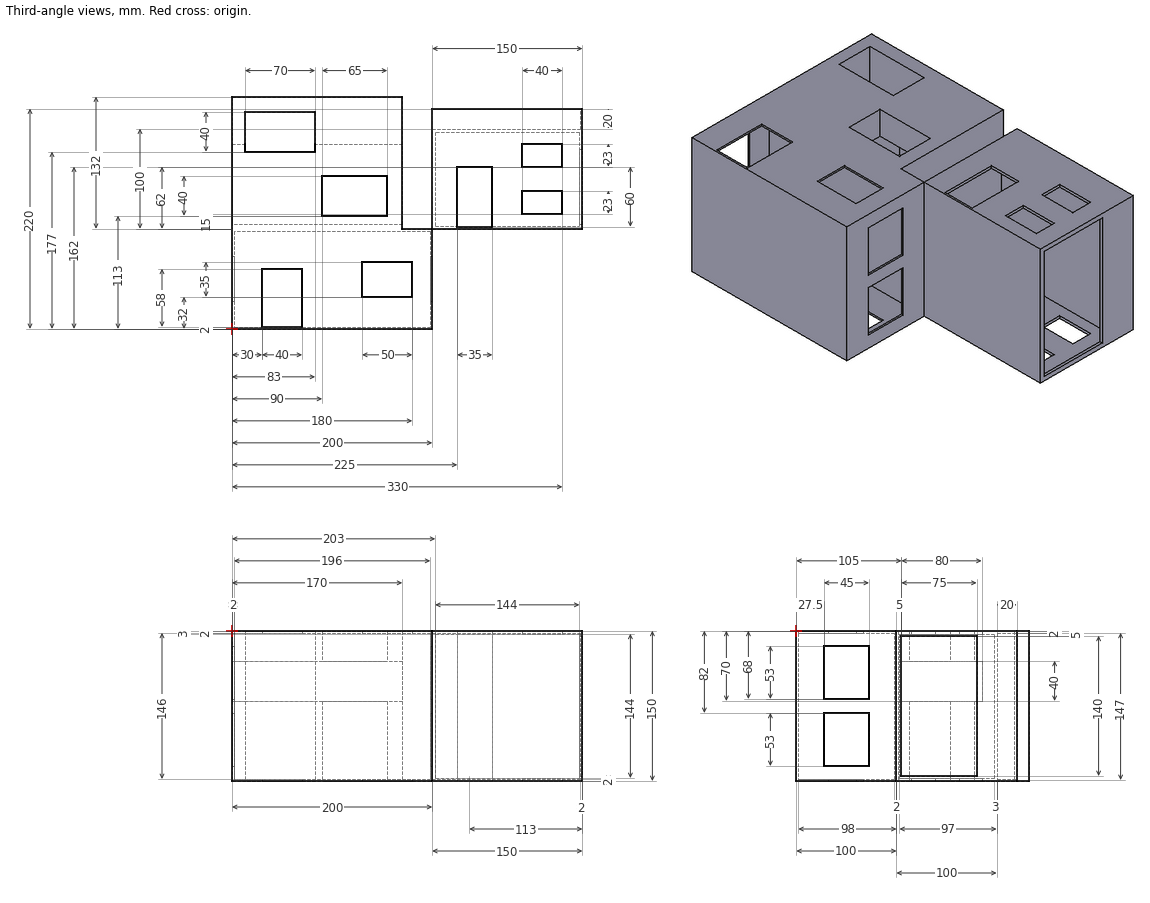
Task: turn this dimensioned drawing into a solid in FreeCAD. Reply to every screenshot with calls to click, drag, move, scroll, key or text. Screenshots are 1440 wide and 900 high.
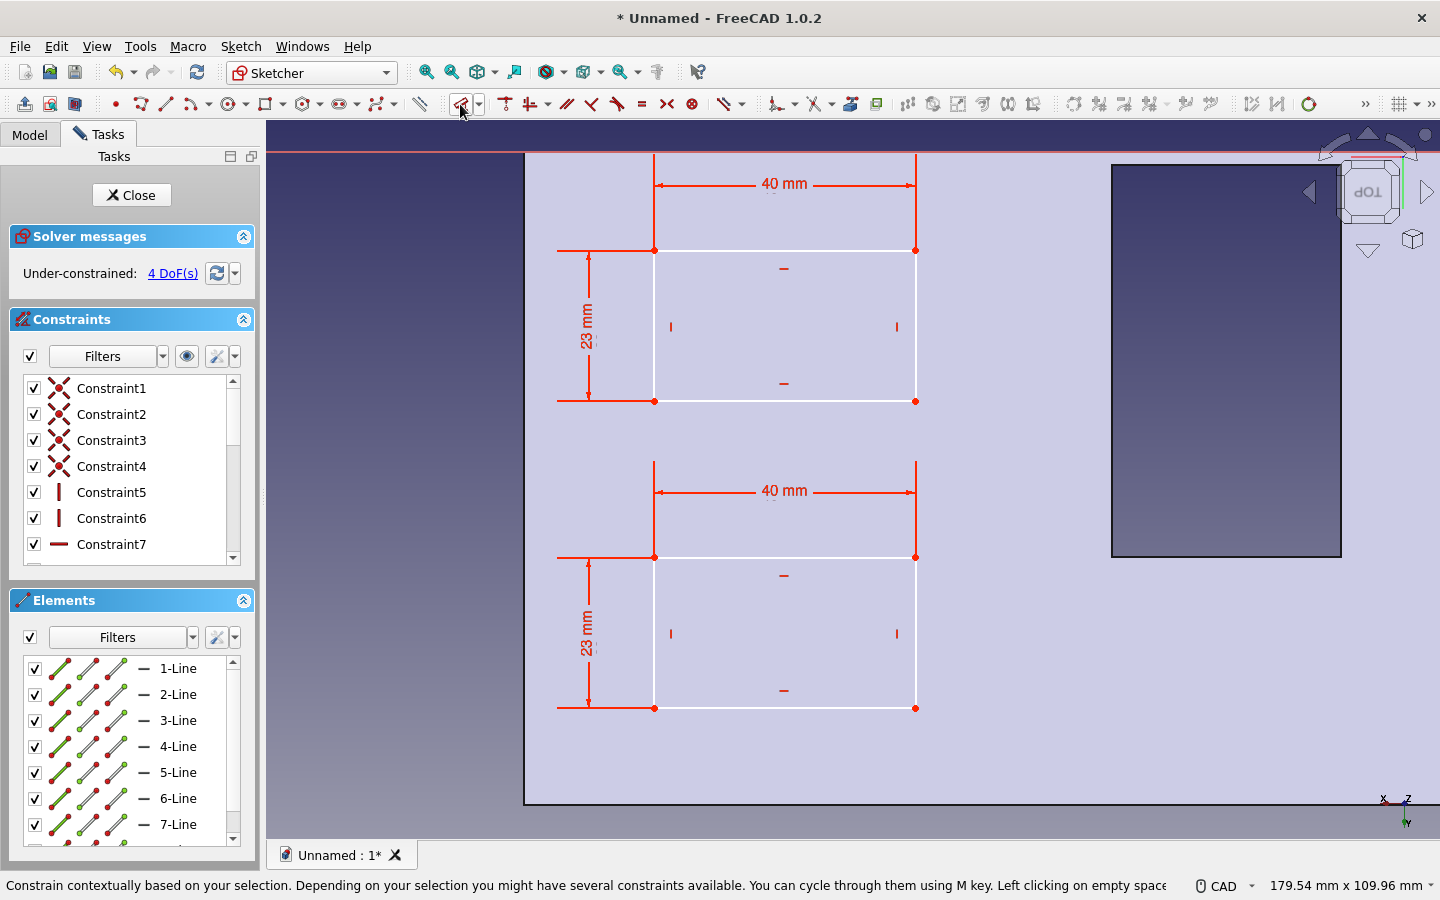
click(654, 251)
click(620, 201)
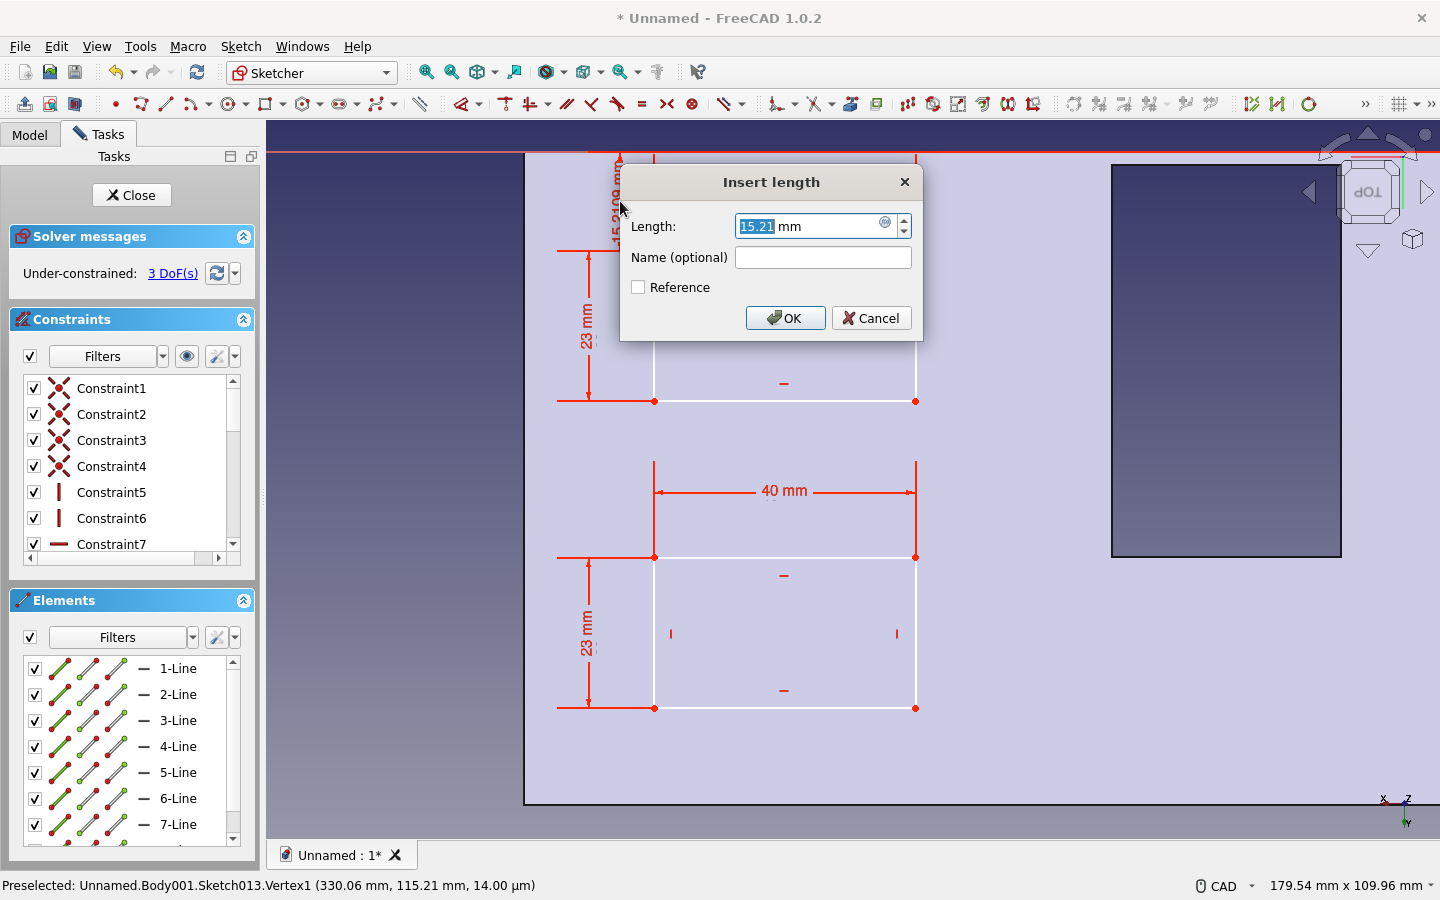
text(15)
key(Return)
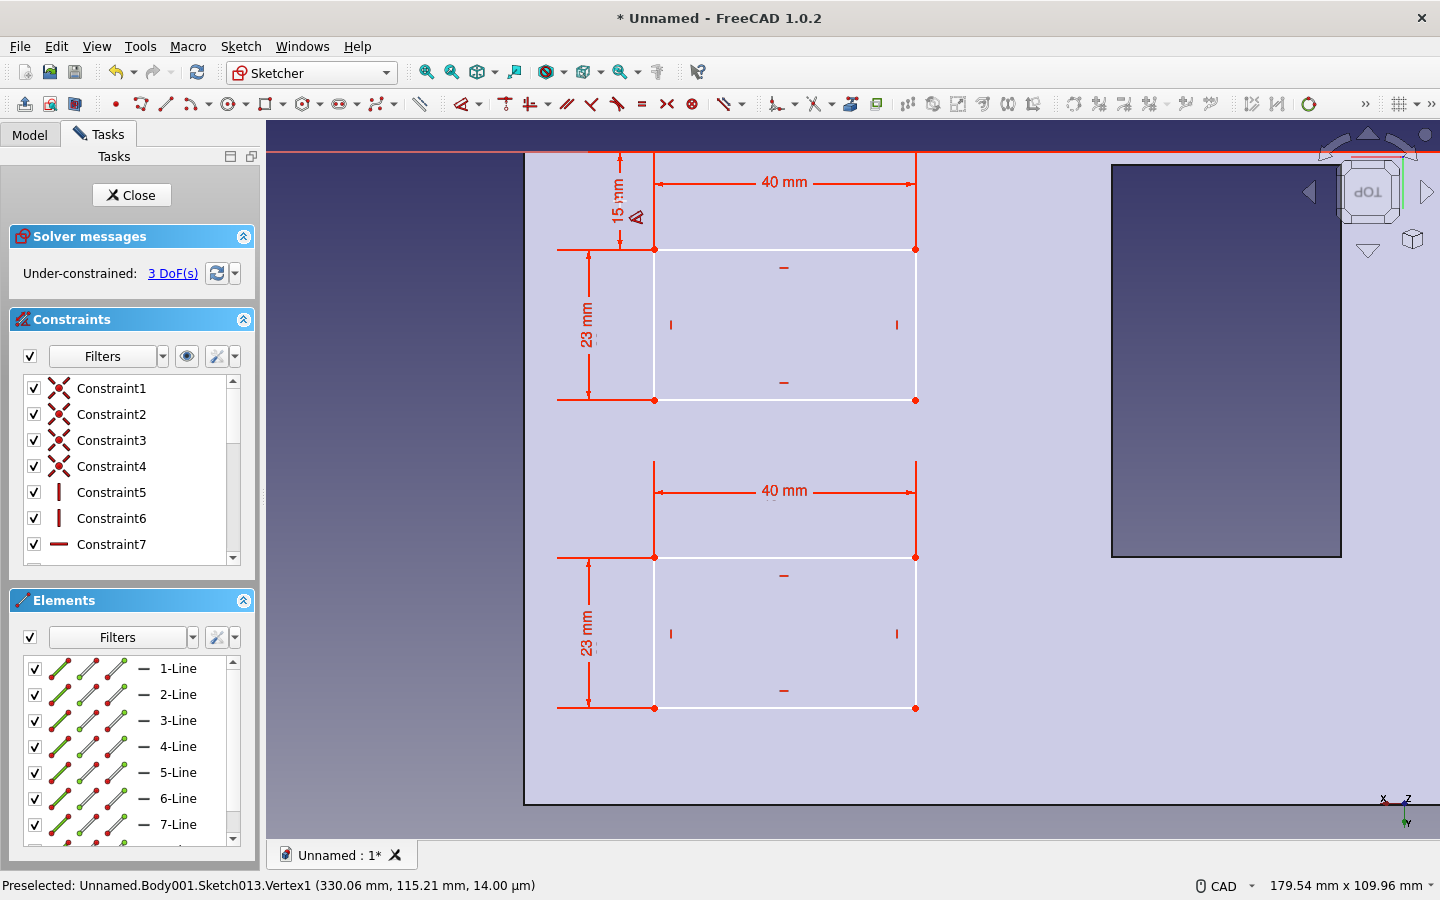
click(654, 558)
click(620, 355)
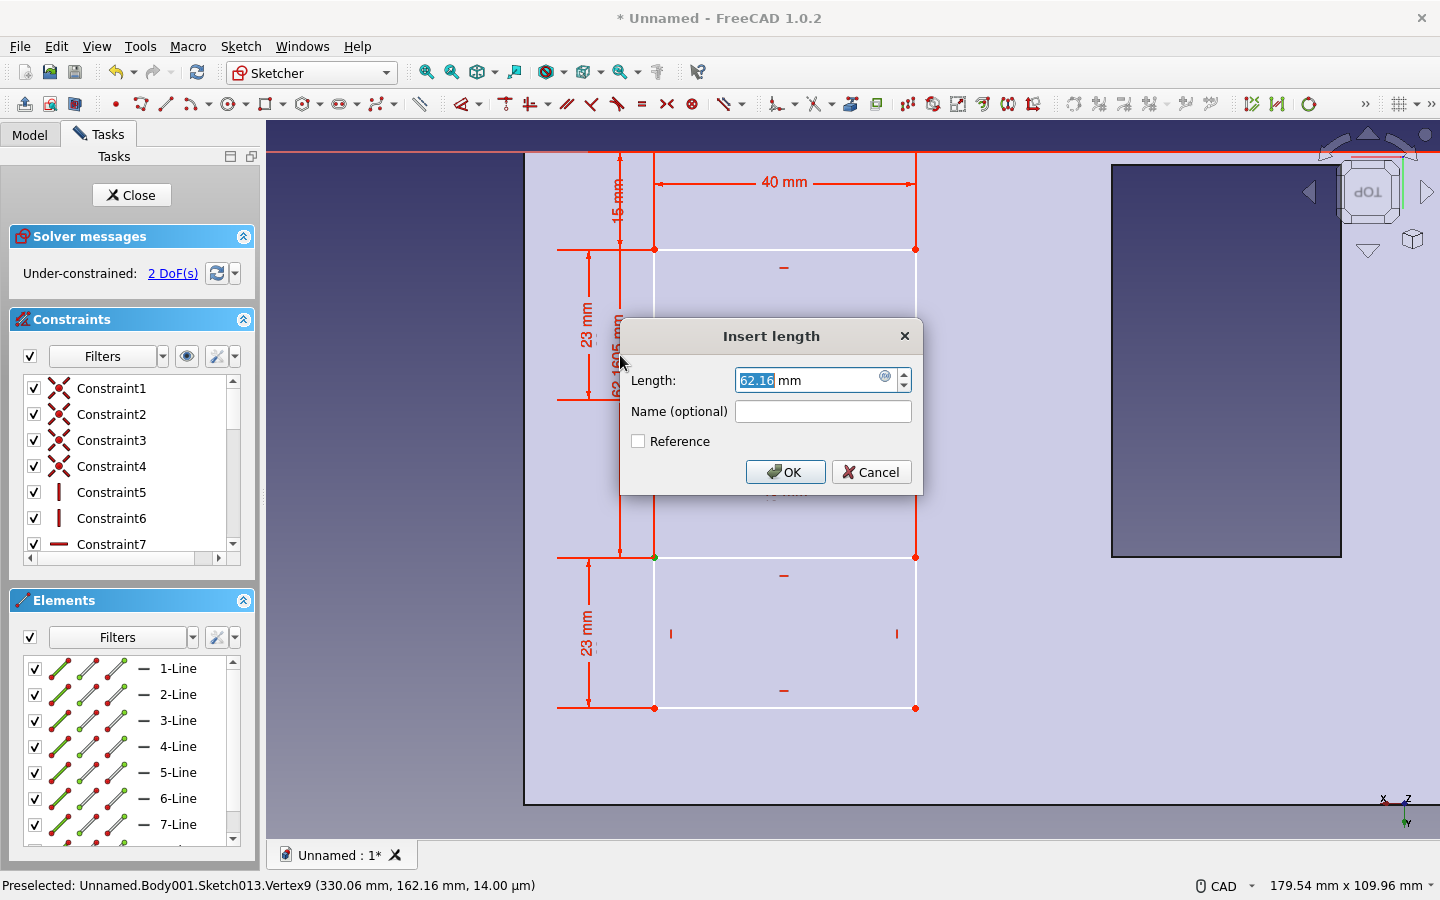
text(62)
key(Return)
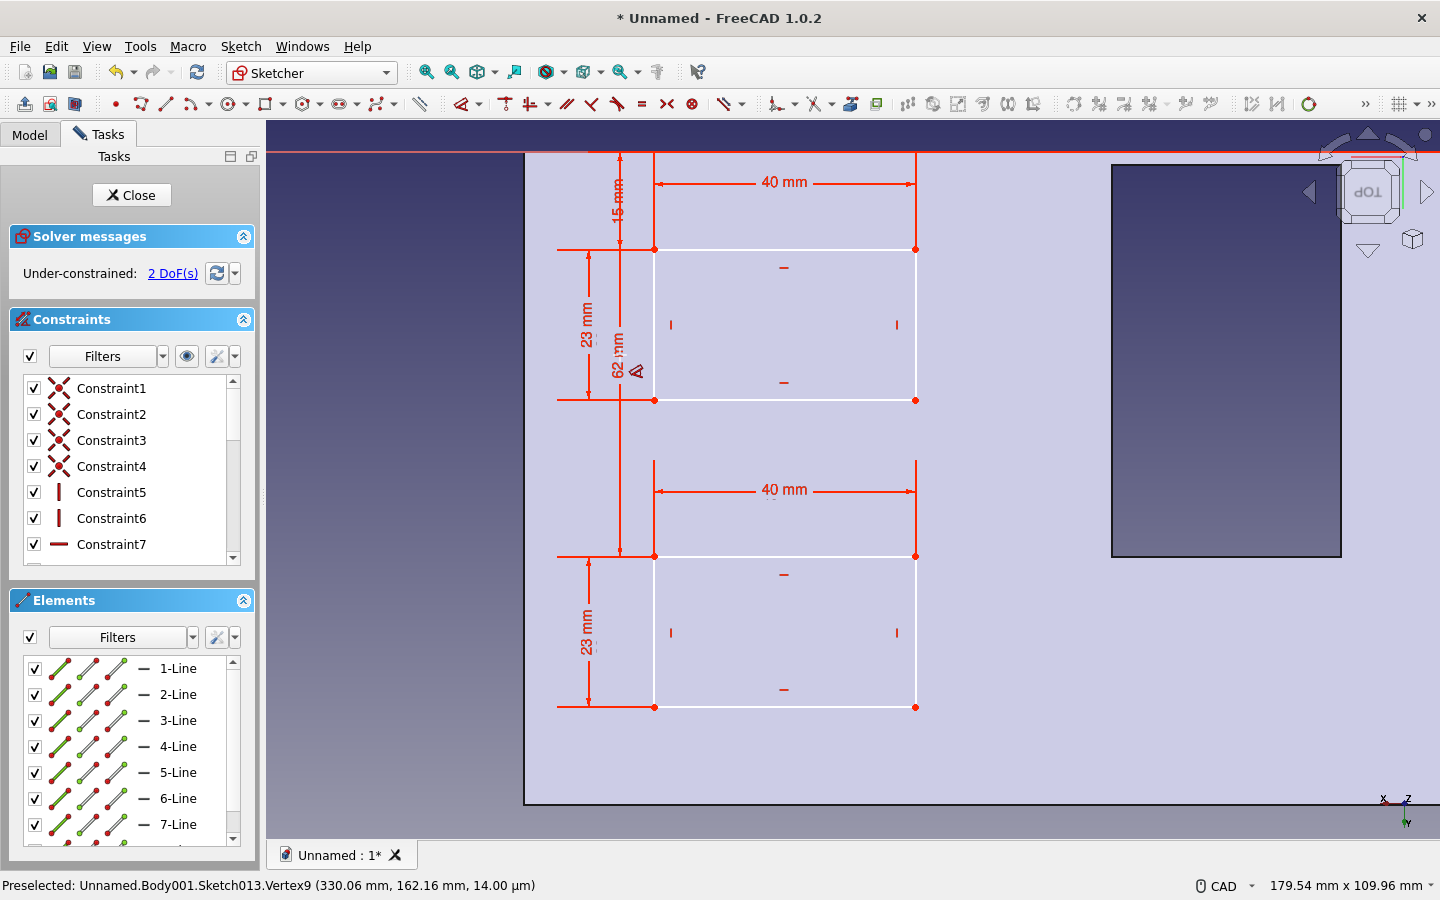
click(654, 250)
click(965, 284)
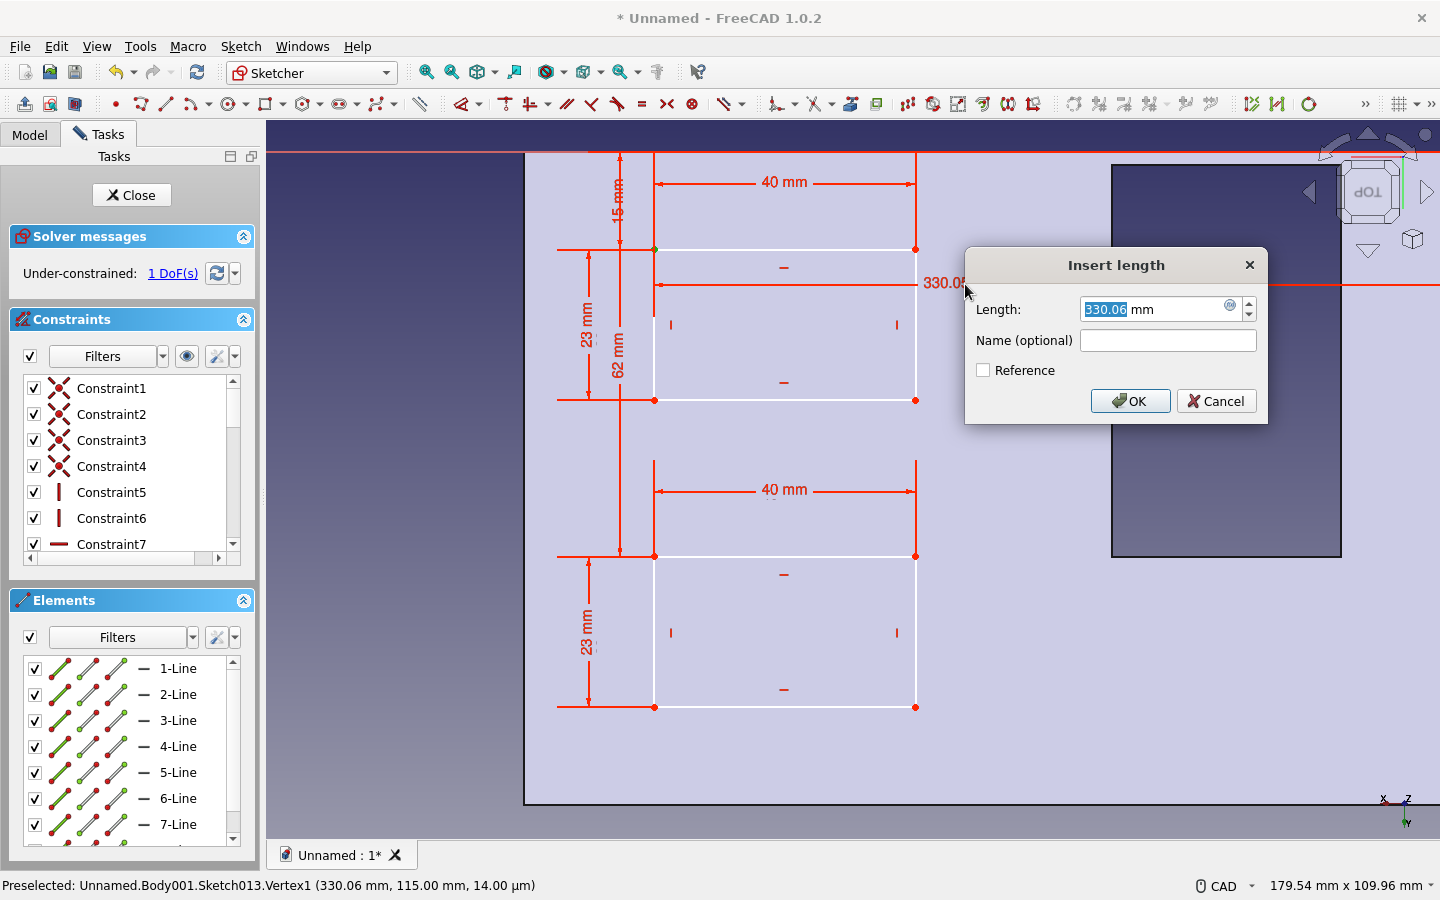
text(330)
key(Return)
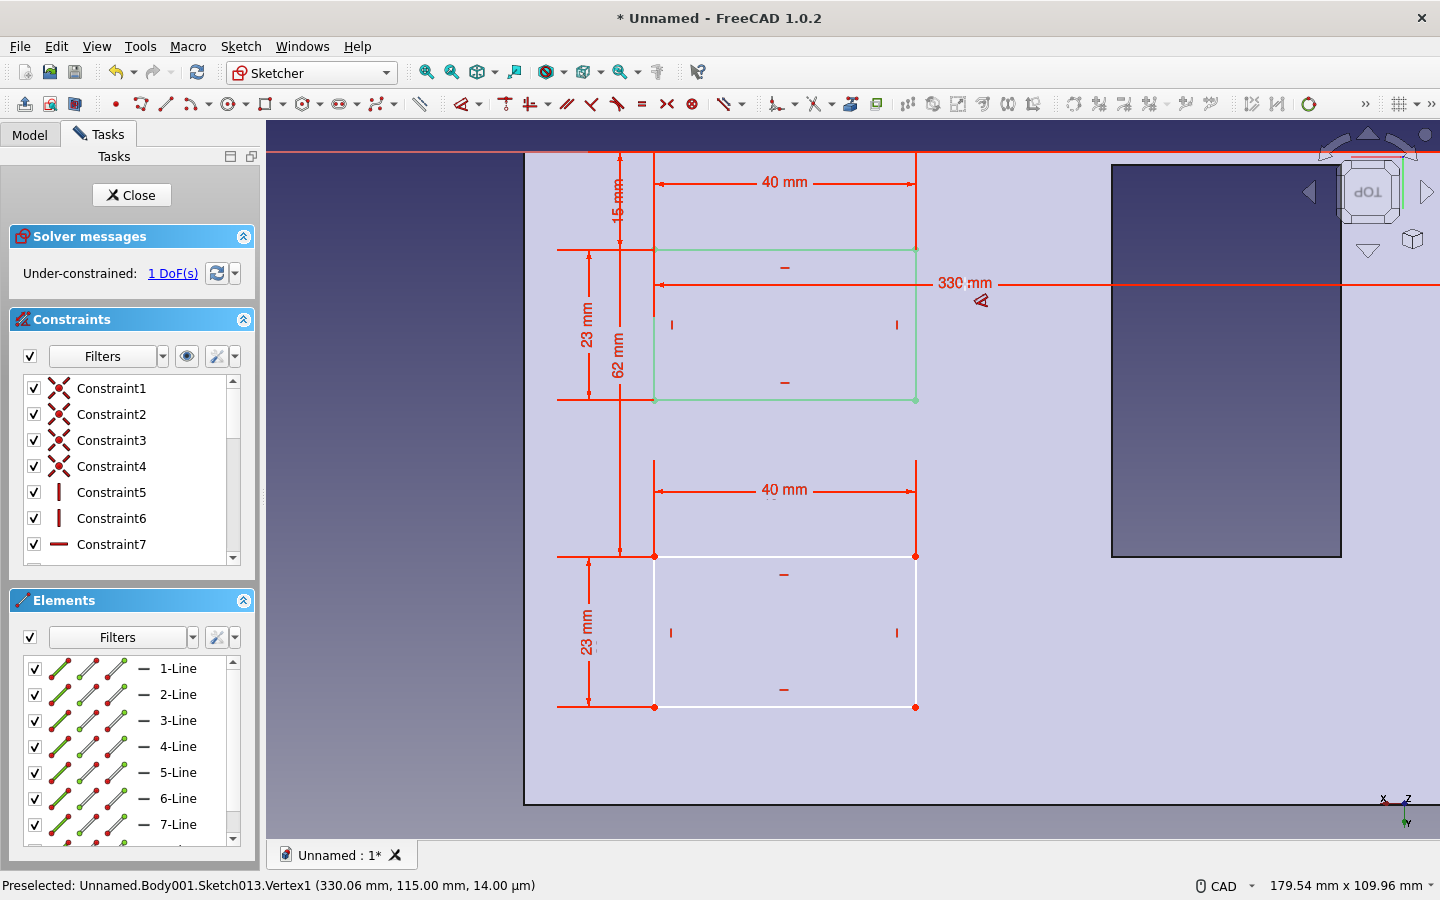
click(654, 557)
click(965, 591)